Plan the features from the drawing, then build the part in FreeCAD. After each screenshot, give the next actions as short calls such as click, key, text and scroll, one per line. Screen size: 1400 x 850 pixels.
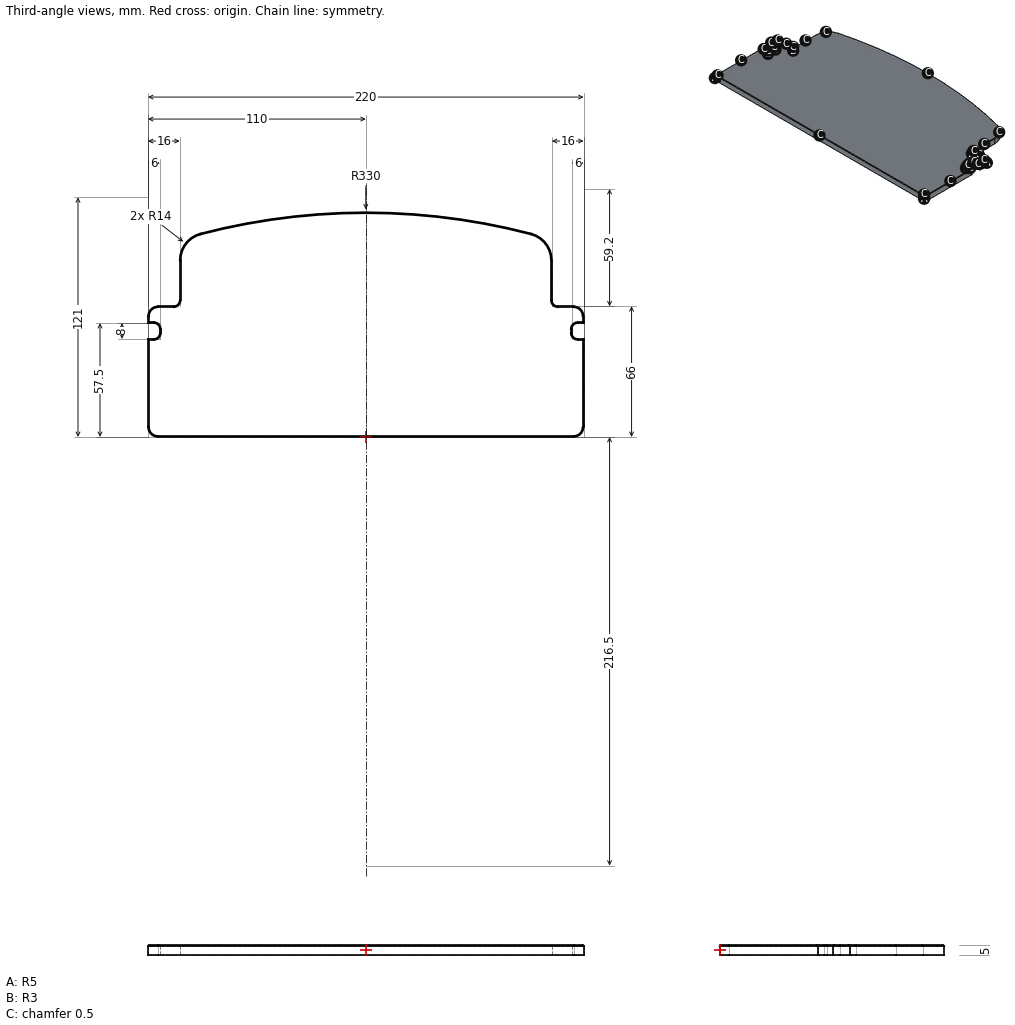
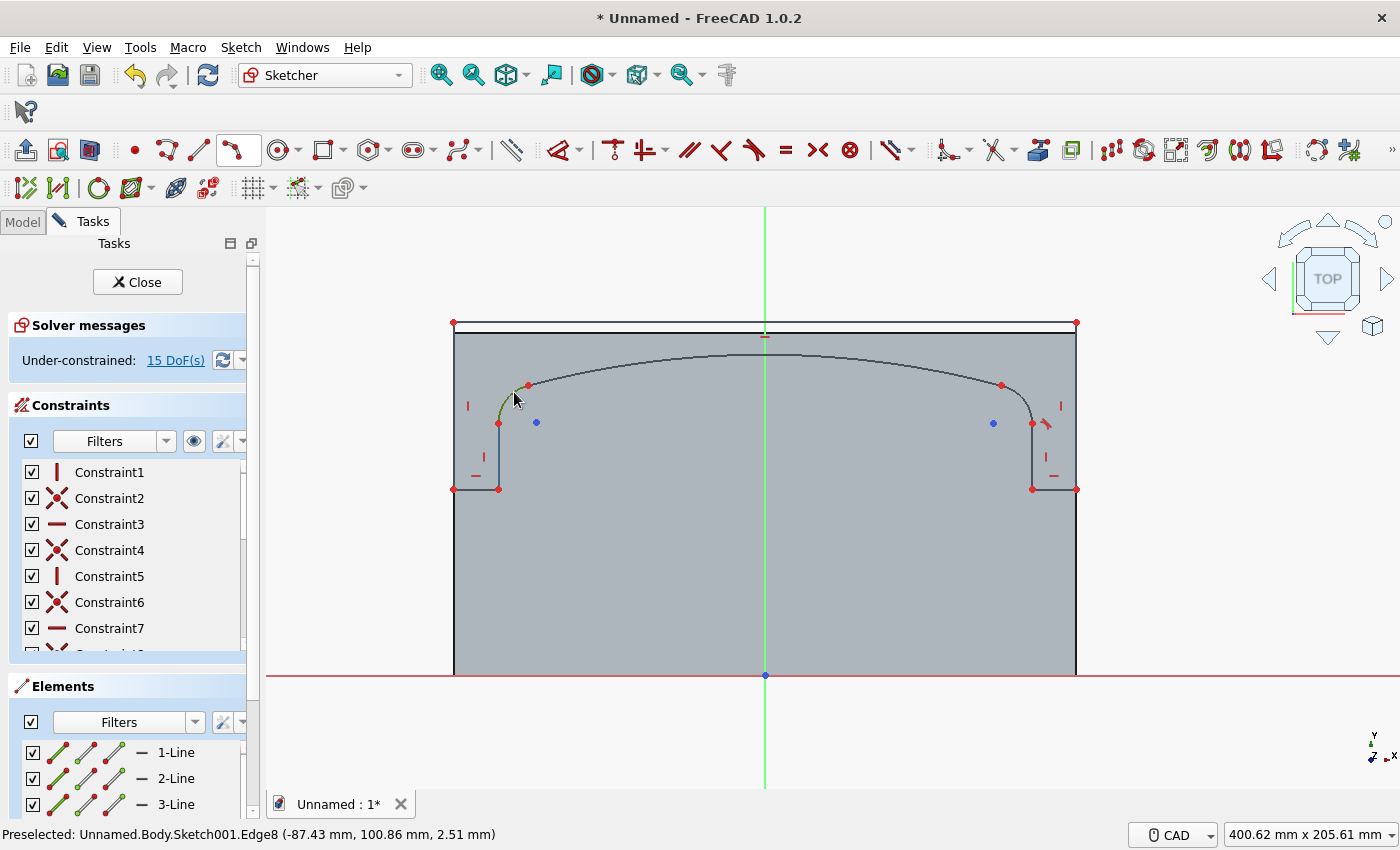
key(t)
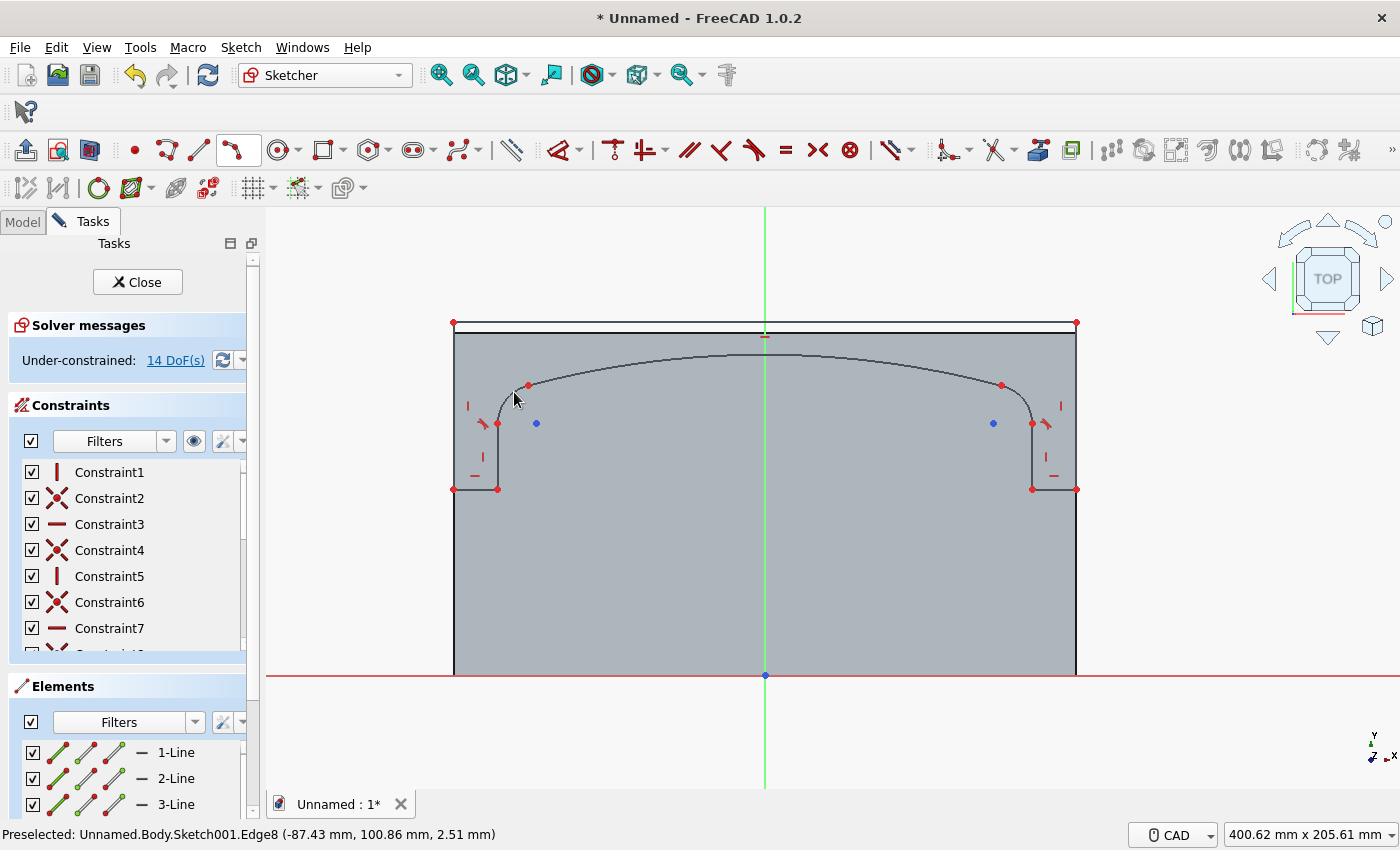
click(514, 392)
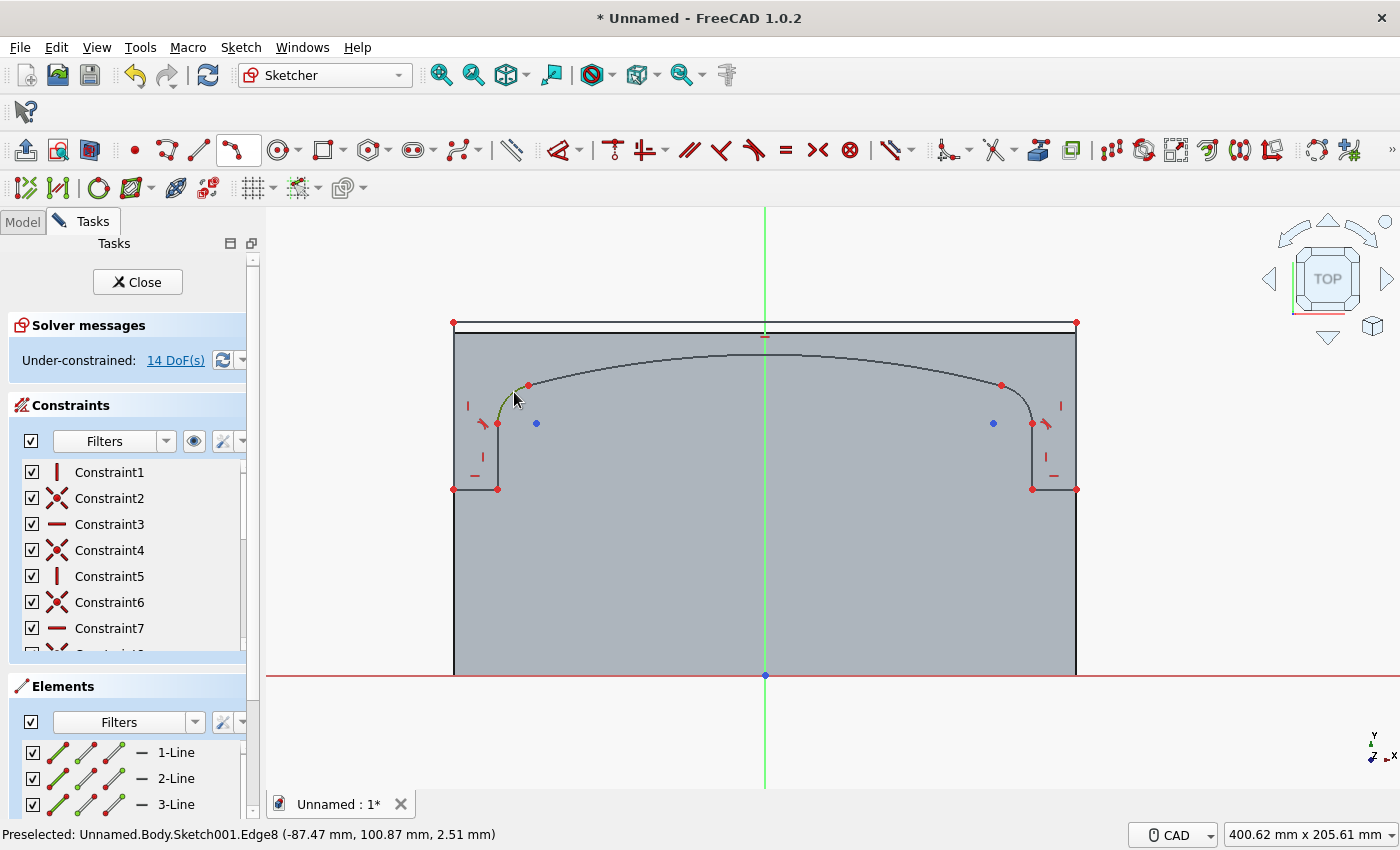
click(860, 360)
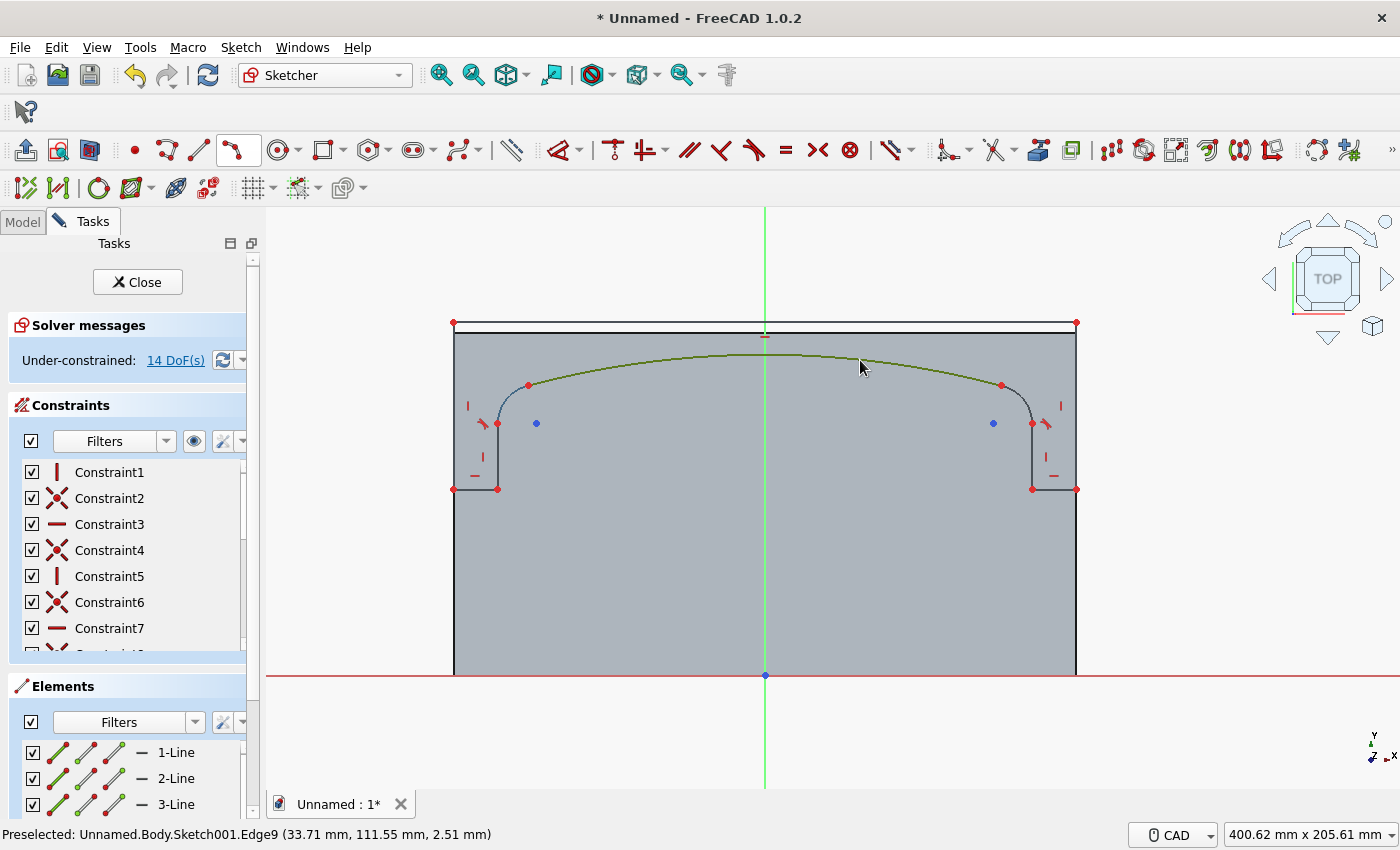
key(t)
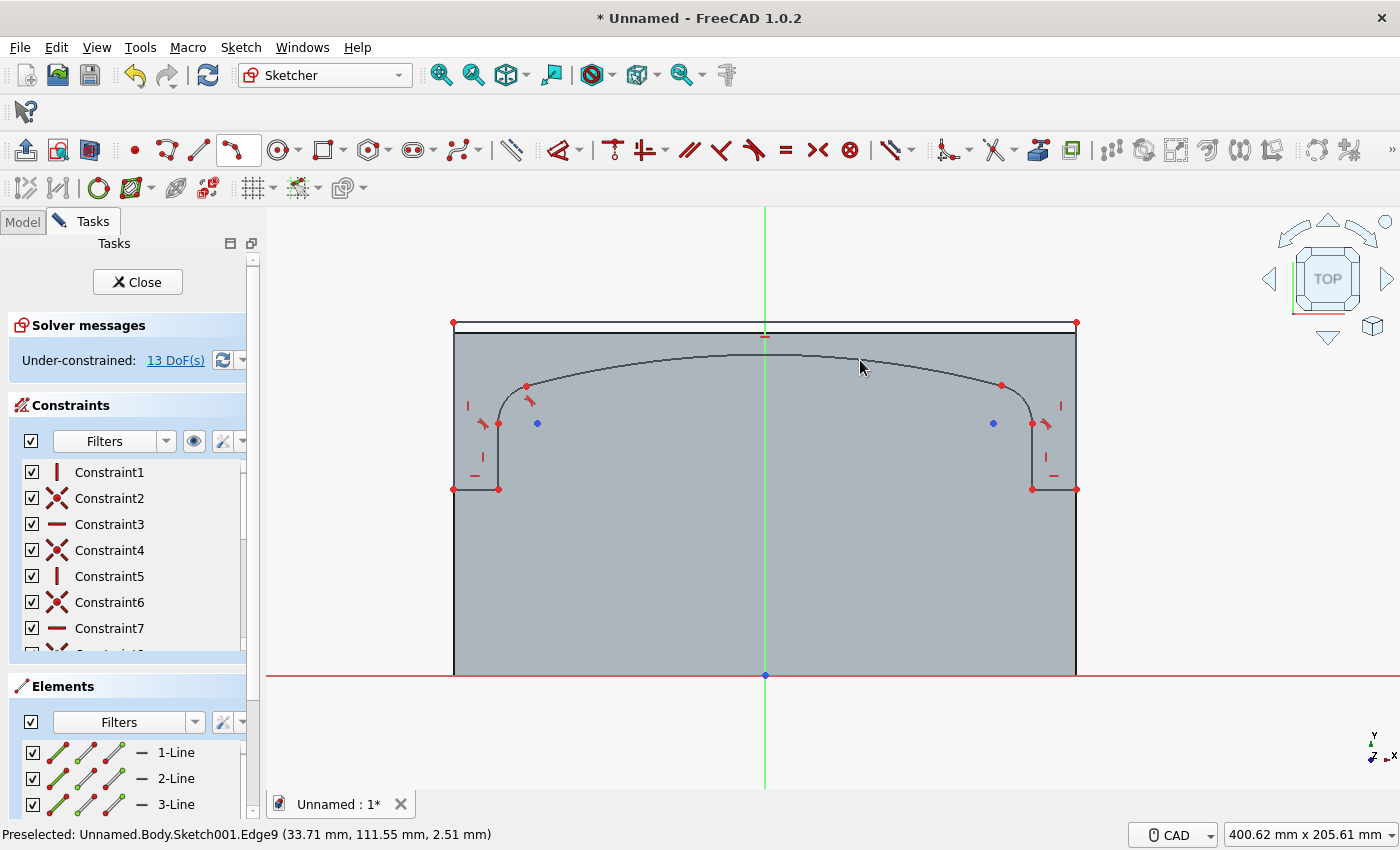
click(860, 360)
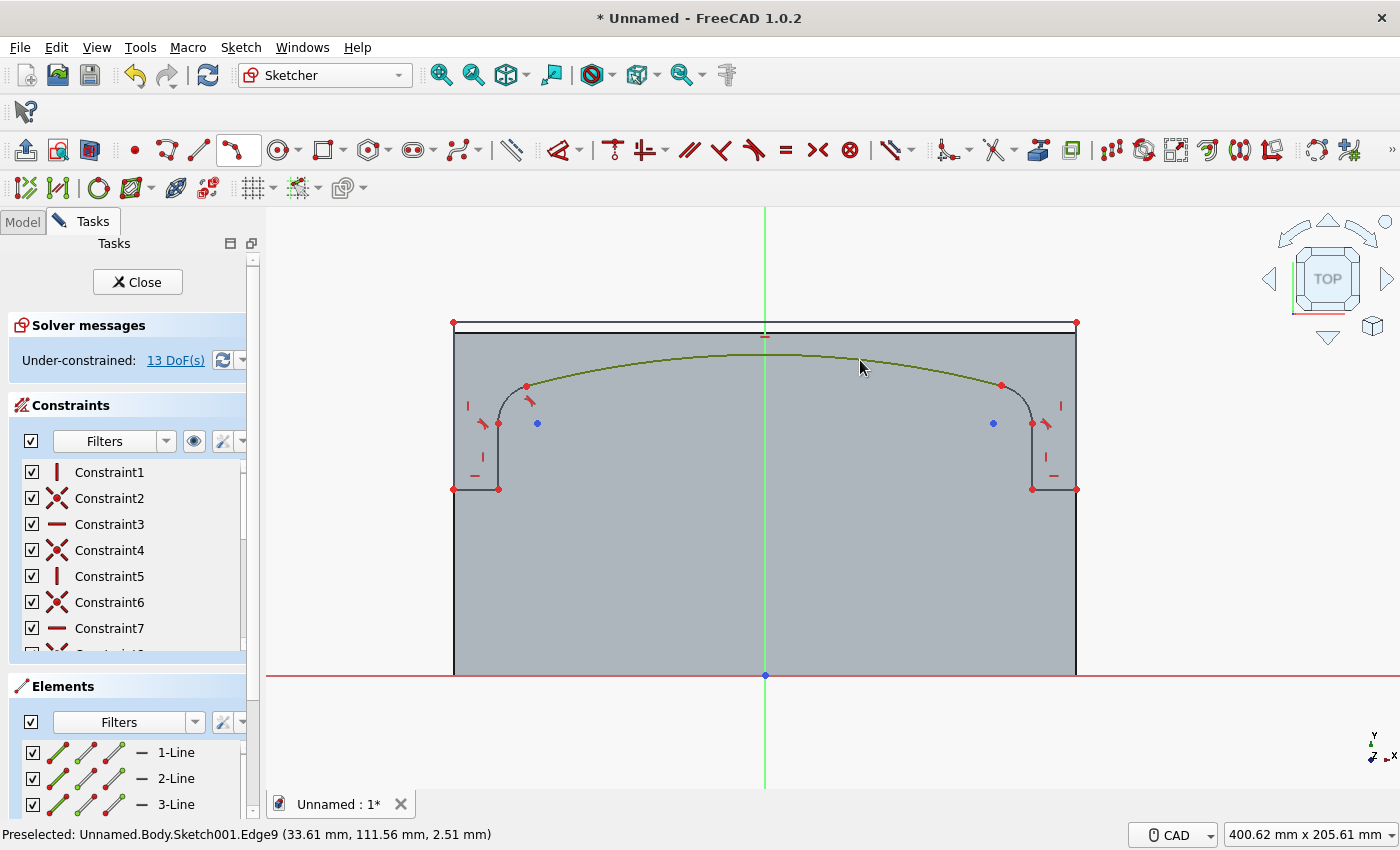
click(1029, 408)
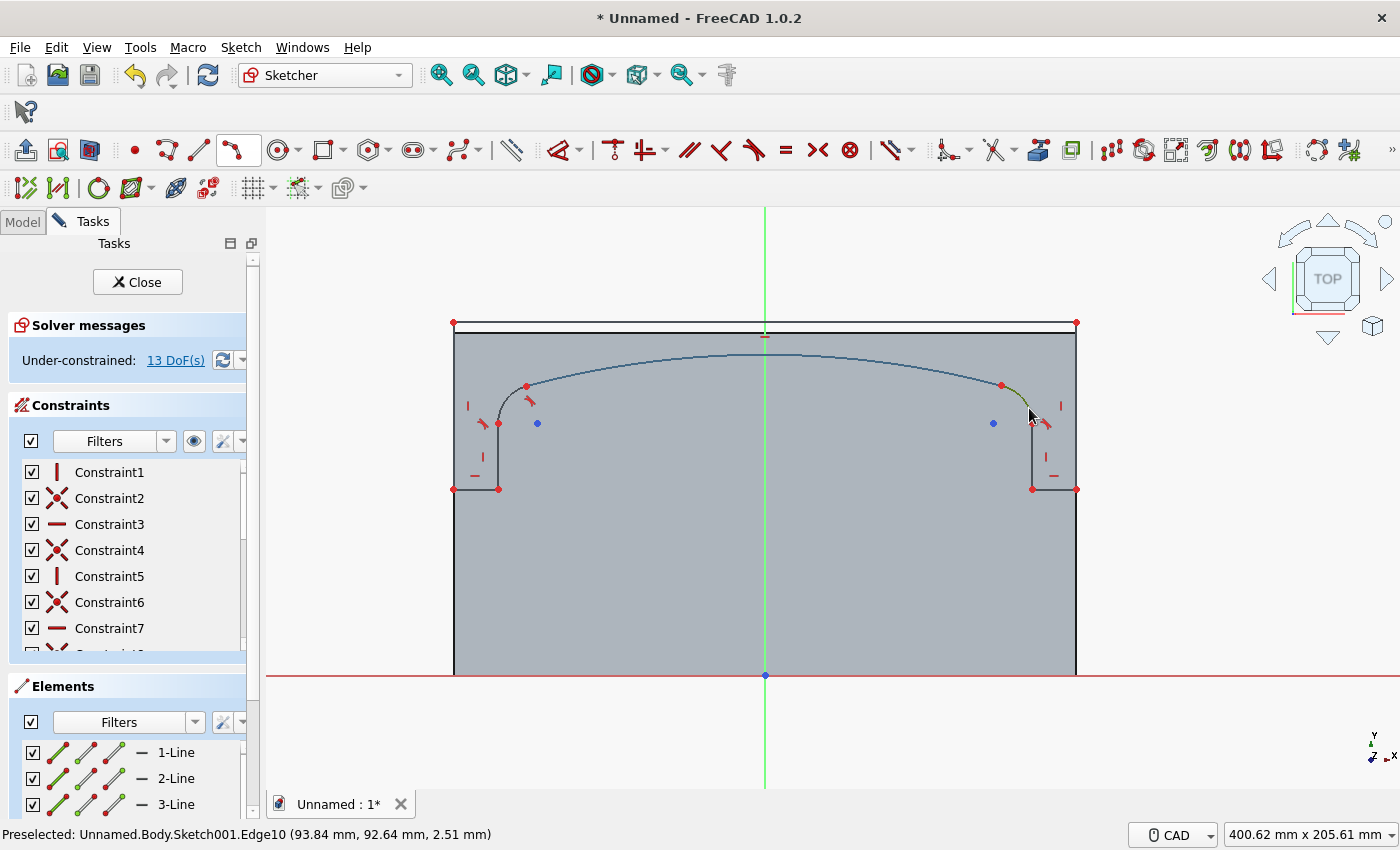
key(t)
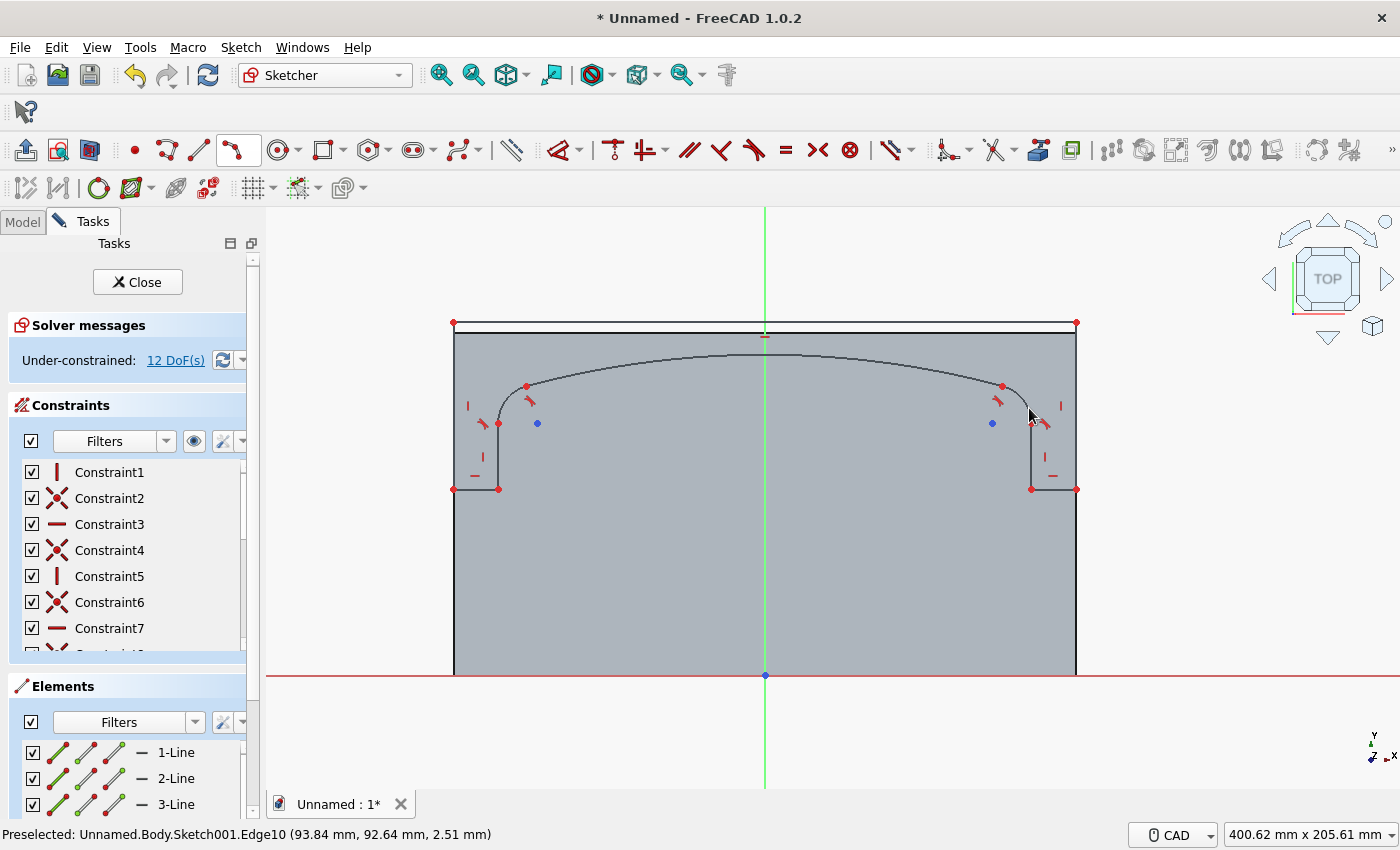
click(513, 393)